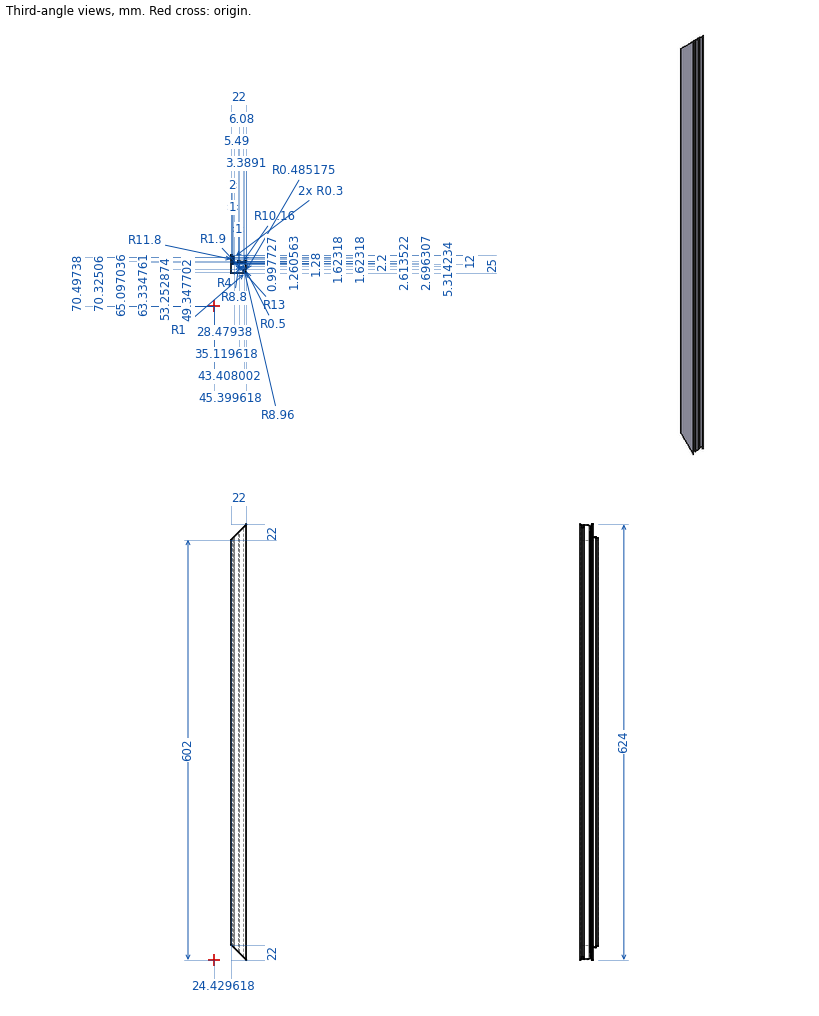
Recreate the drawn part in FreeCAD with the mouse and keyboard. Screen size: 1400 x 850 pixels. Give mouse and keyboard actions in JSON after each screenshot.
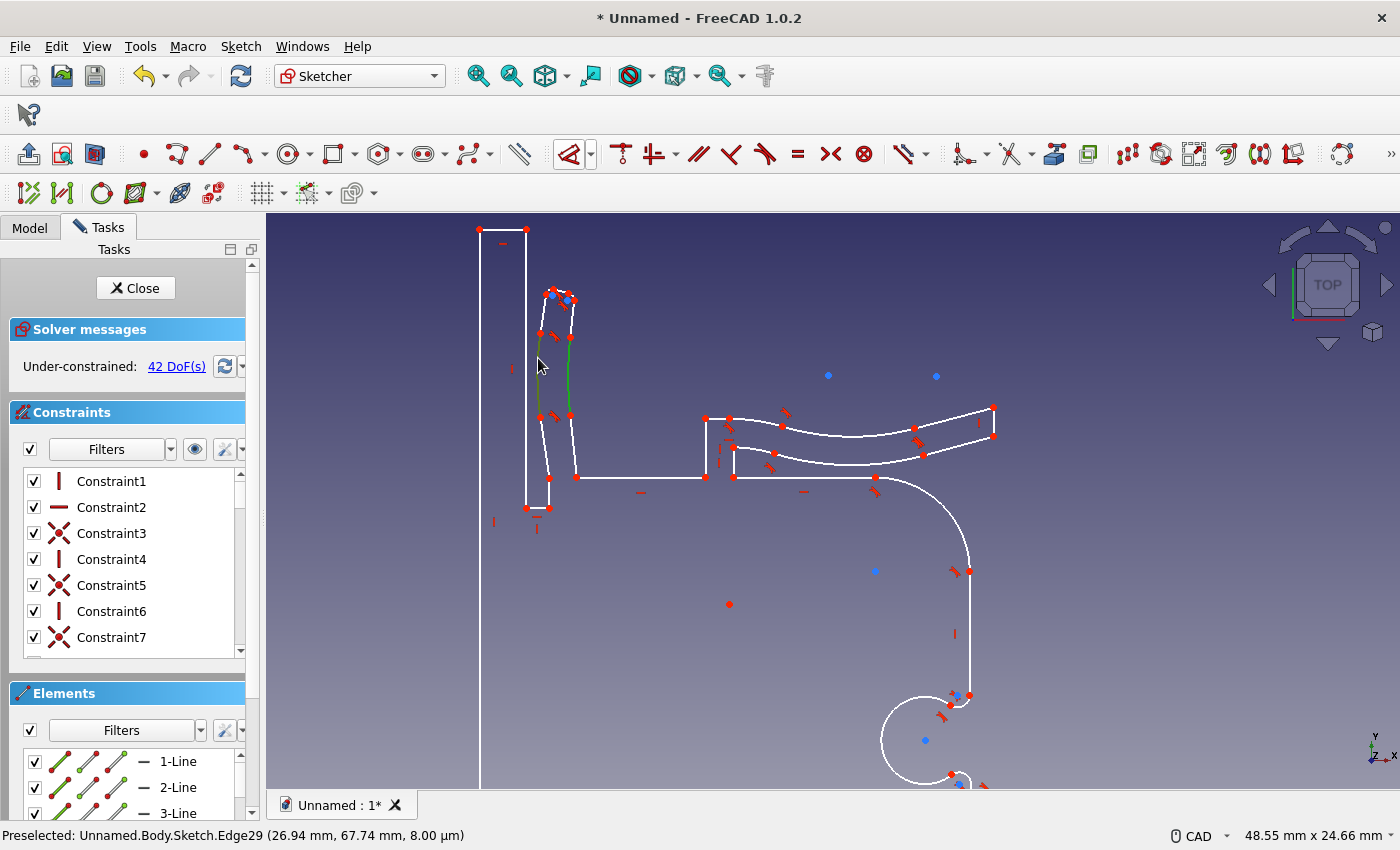
{"action": "key", "text": "c"}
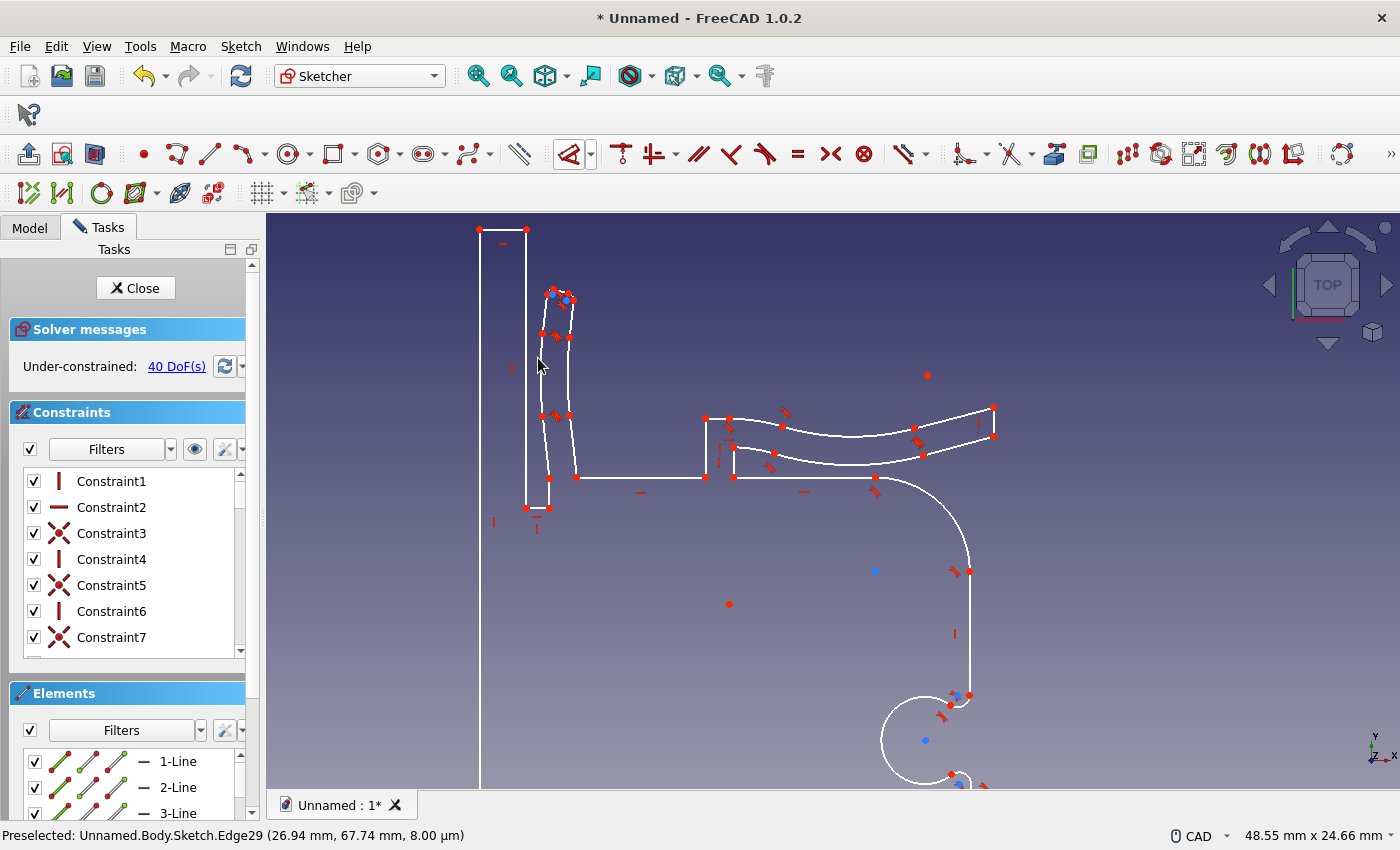
{"action": "scroll", "coordinate": [572, 296], "scroll_direction": "up", "scroll_amount": 6}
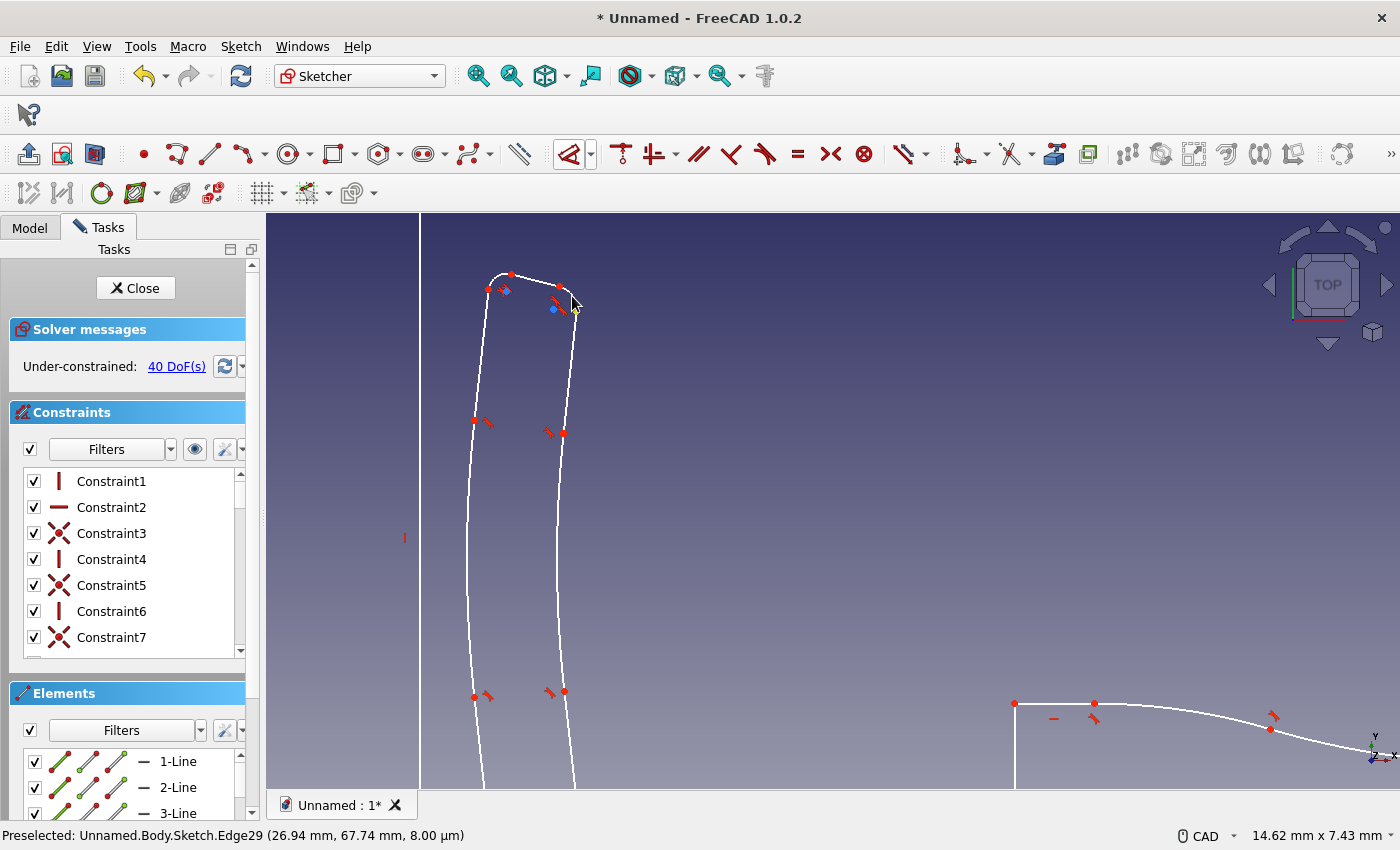
{"action": "left_click", "coordinate": [573, 296]}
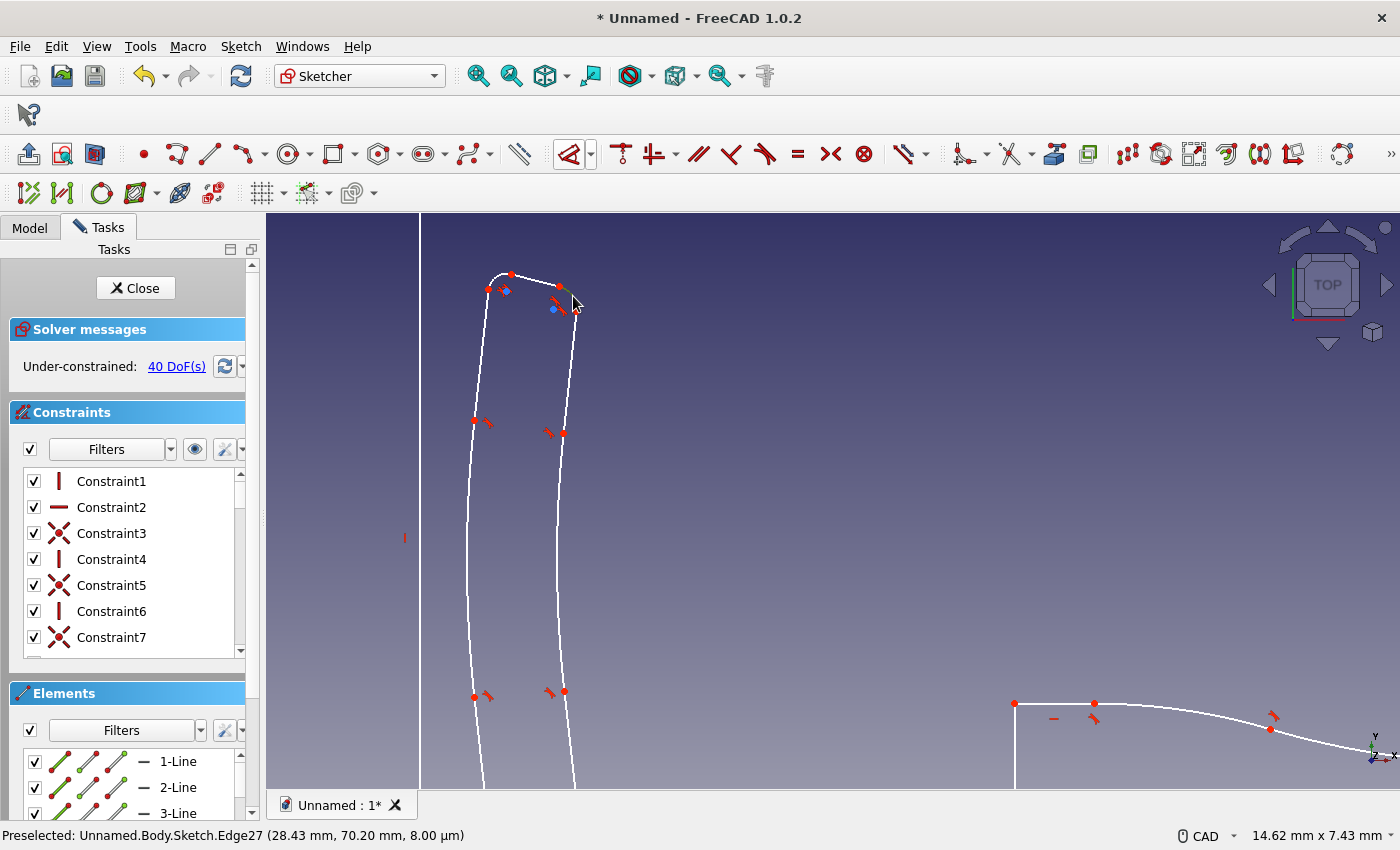
{"action": "scroll", "coordinate": [502, 274], "scroll_direction": "up", "scroll_amount": 3}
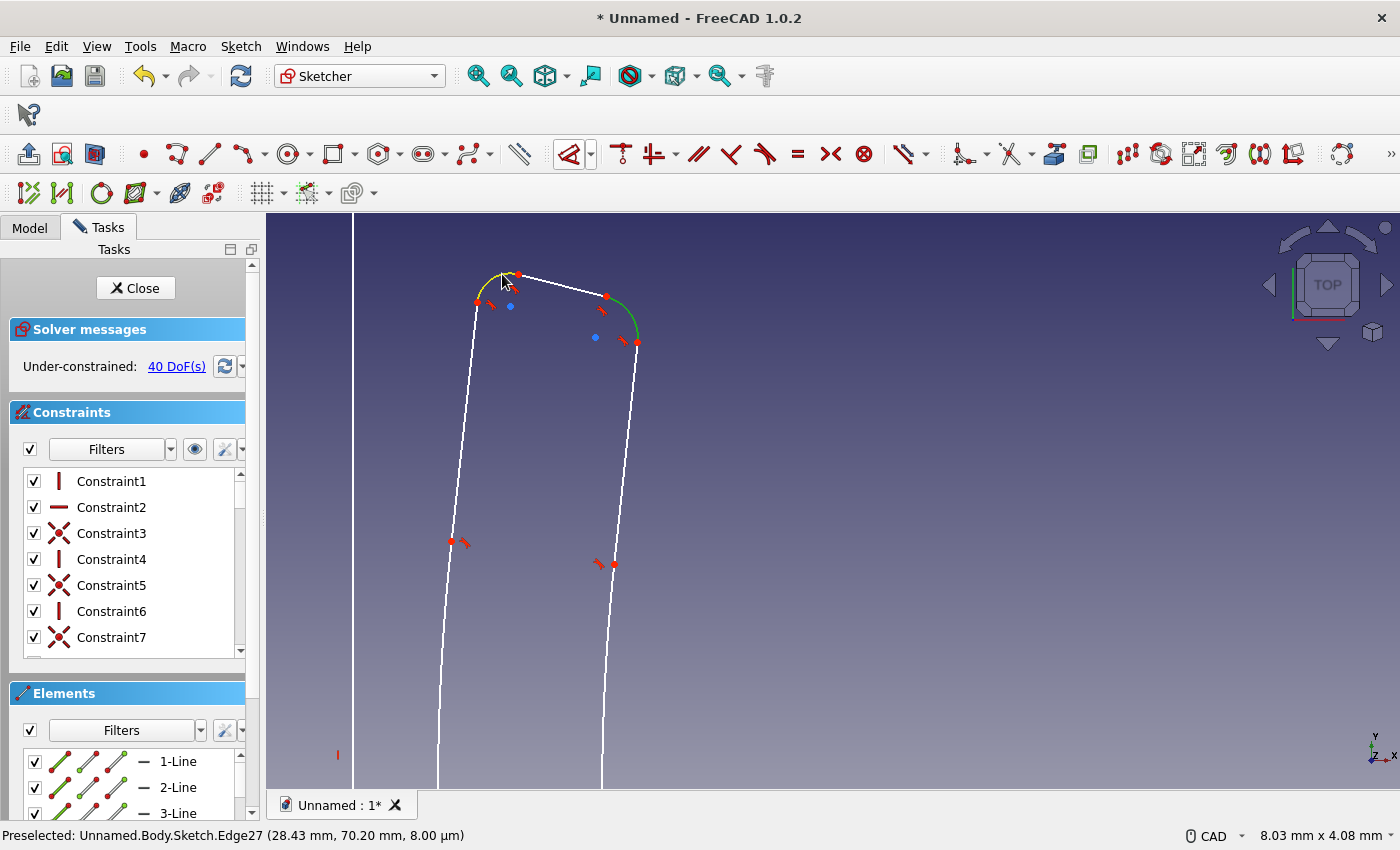
{"action": "left_click", "coordinate": [502, 275]}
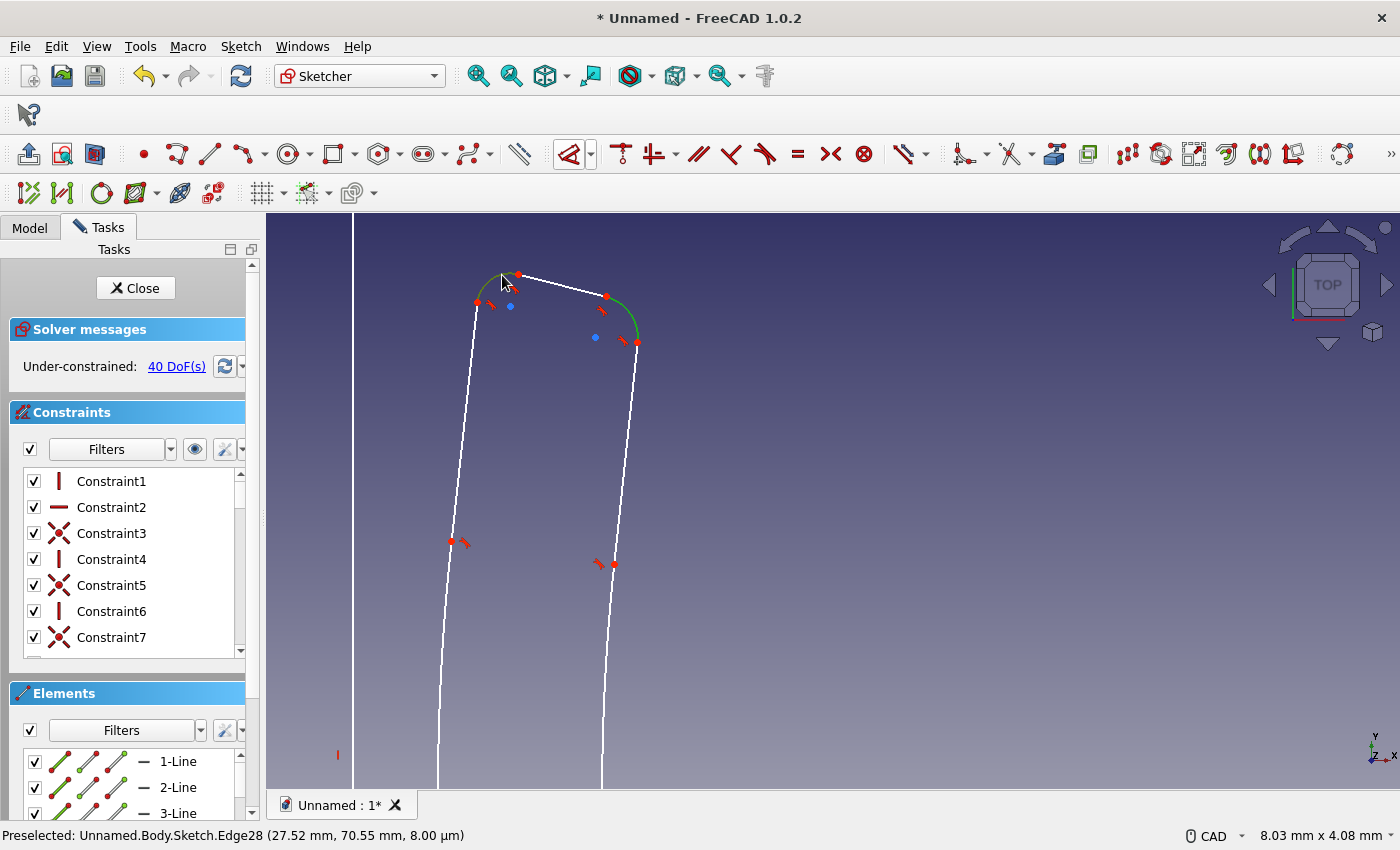
{"action": "key", "text": "e"}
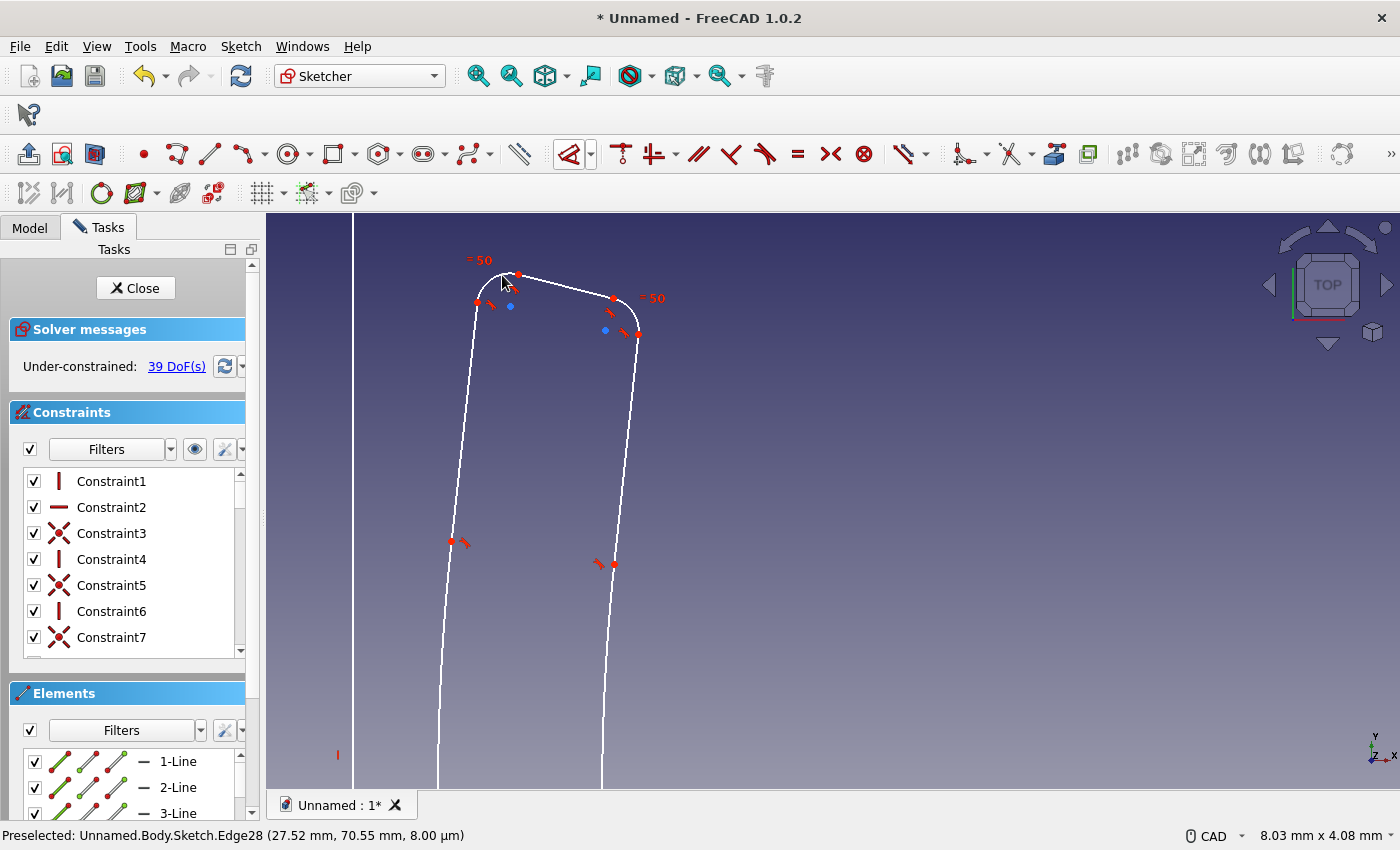
{"action": "left_click", "coordinate": [568, 154]}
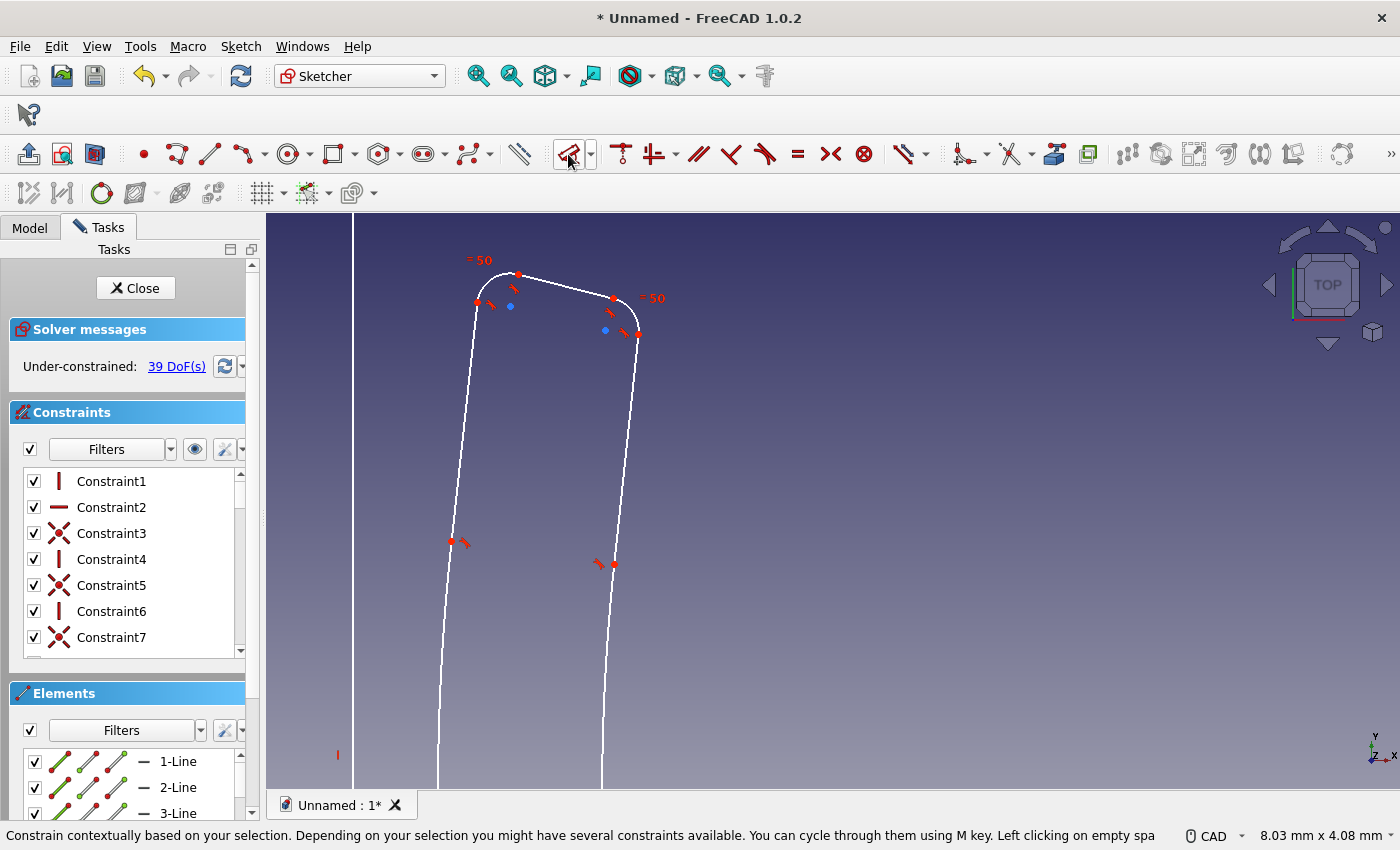
{"action": "scroll", "coordinate": [657, 356], "scroll_direction": "down", "scroll_amount": 11}